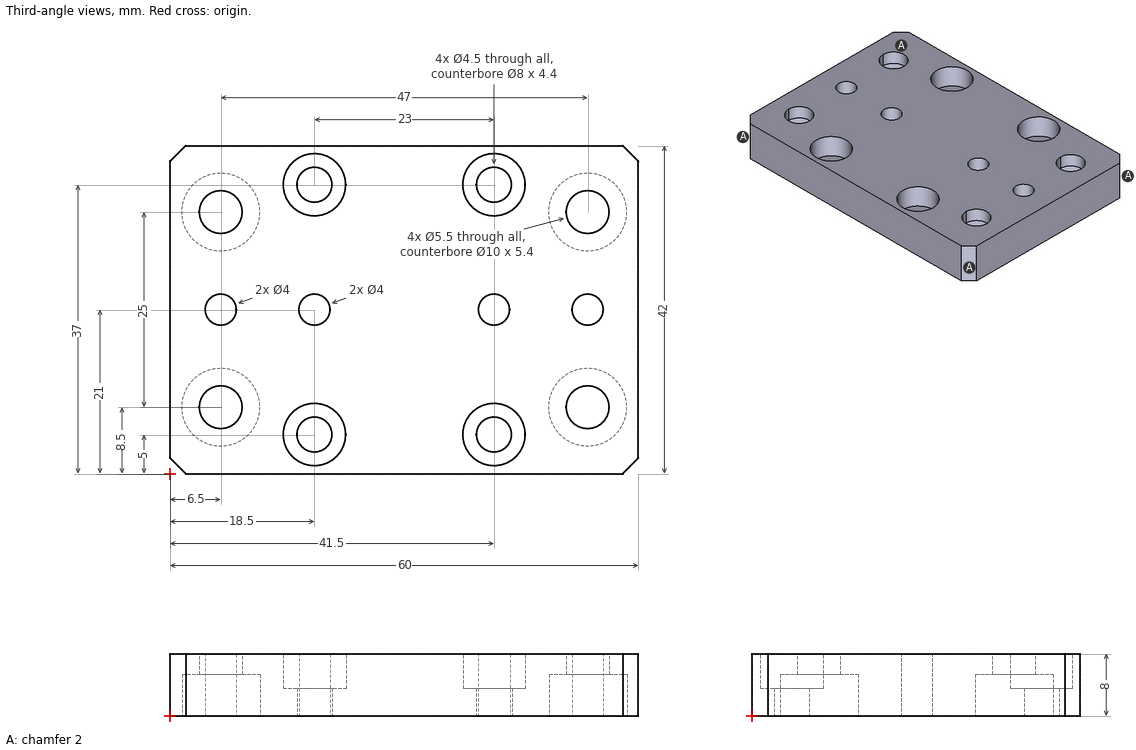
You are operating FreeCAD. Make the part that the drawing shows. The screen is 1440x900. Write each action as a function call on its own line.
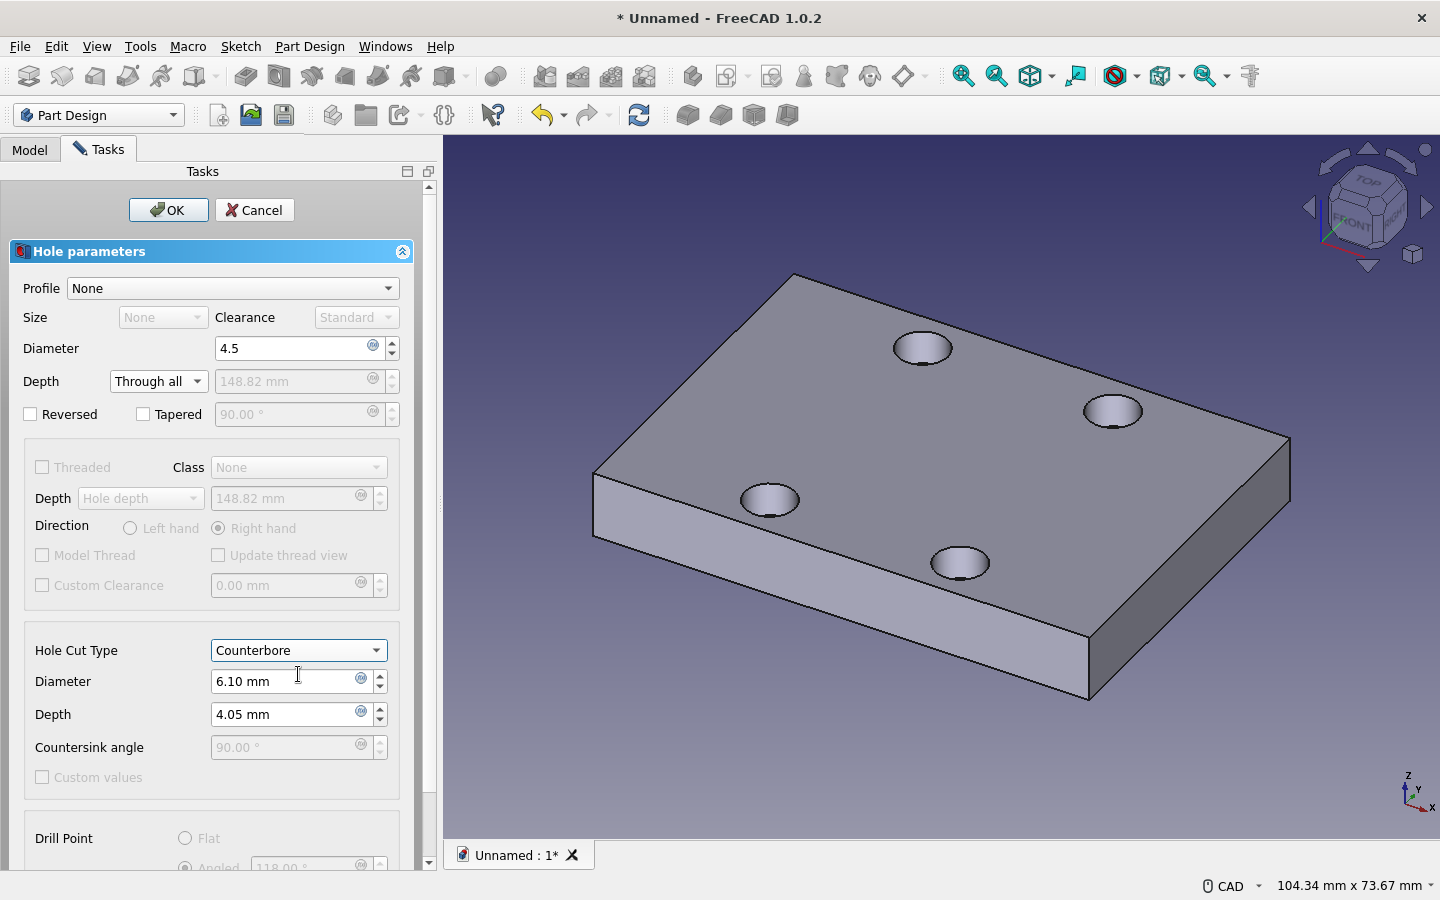
triple_click(292, 682)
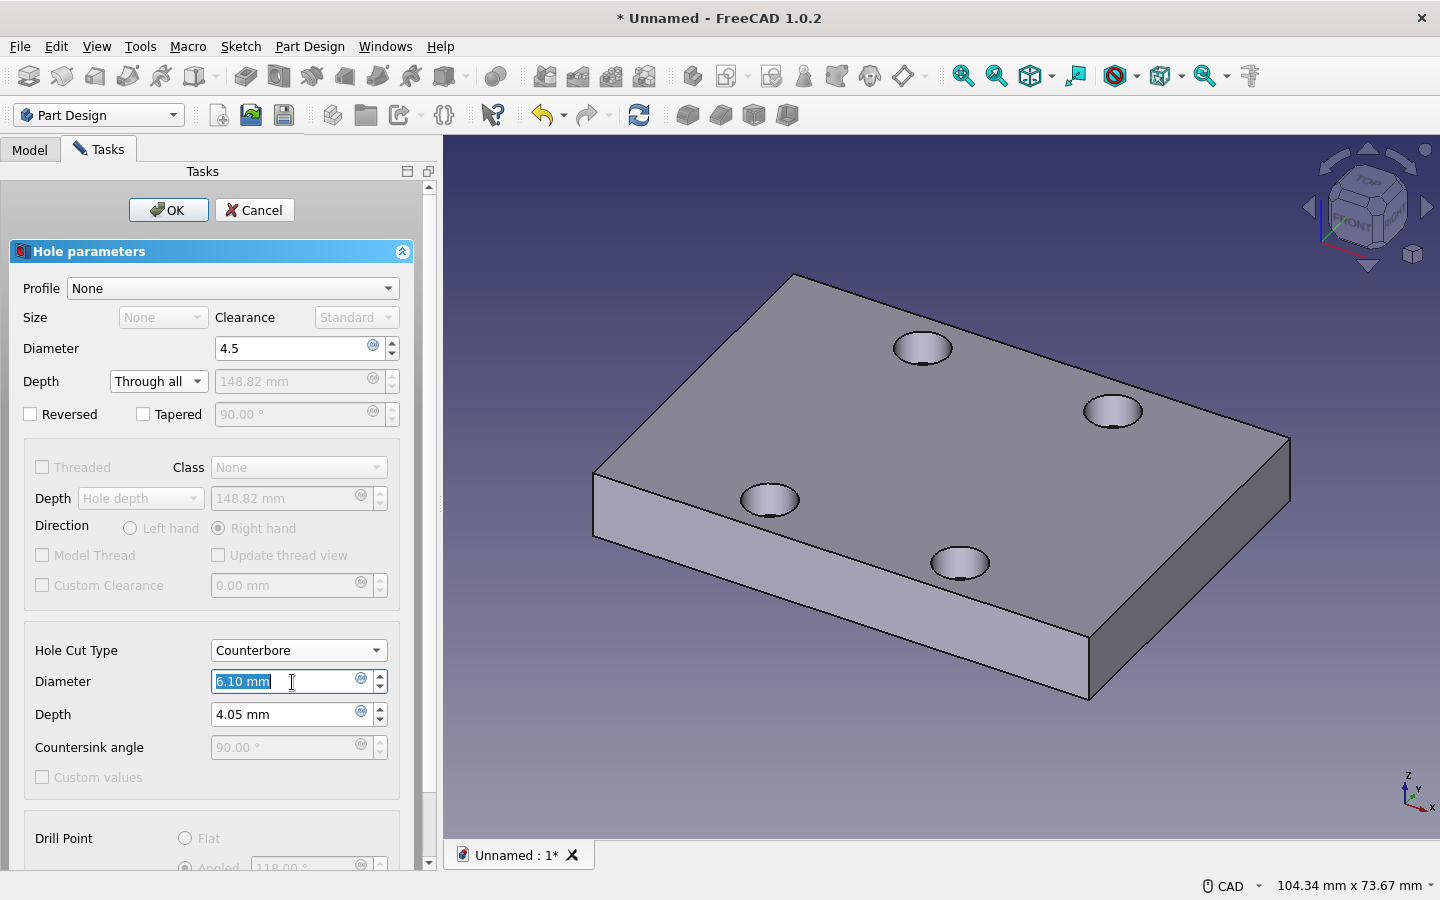
text(8)
key(Tab)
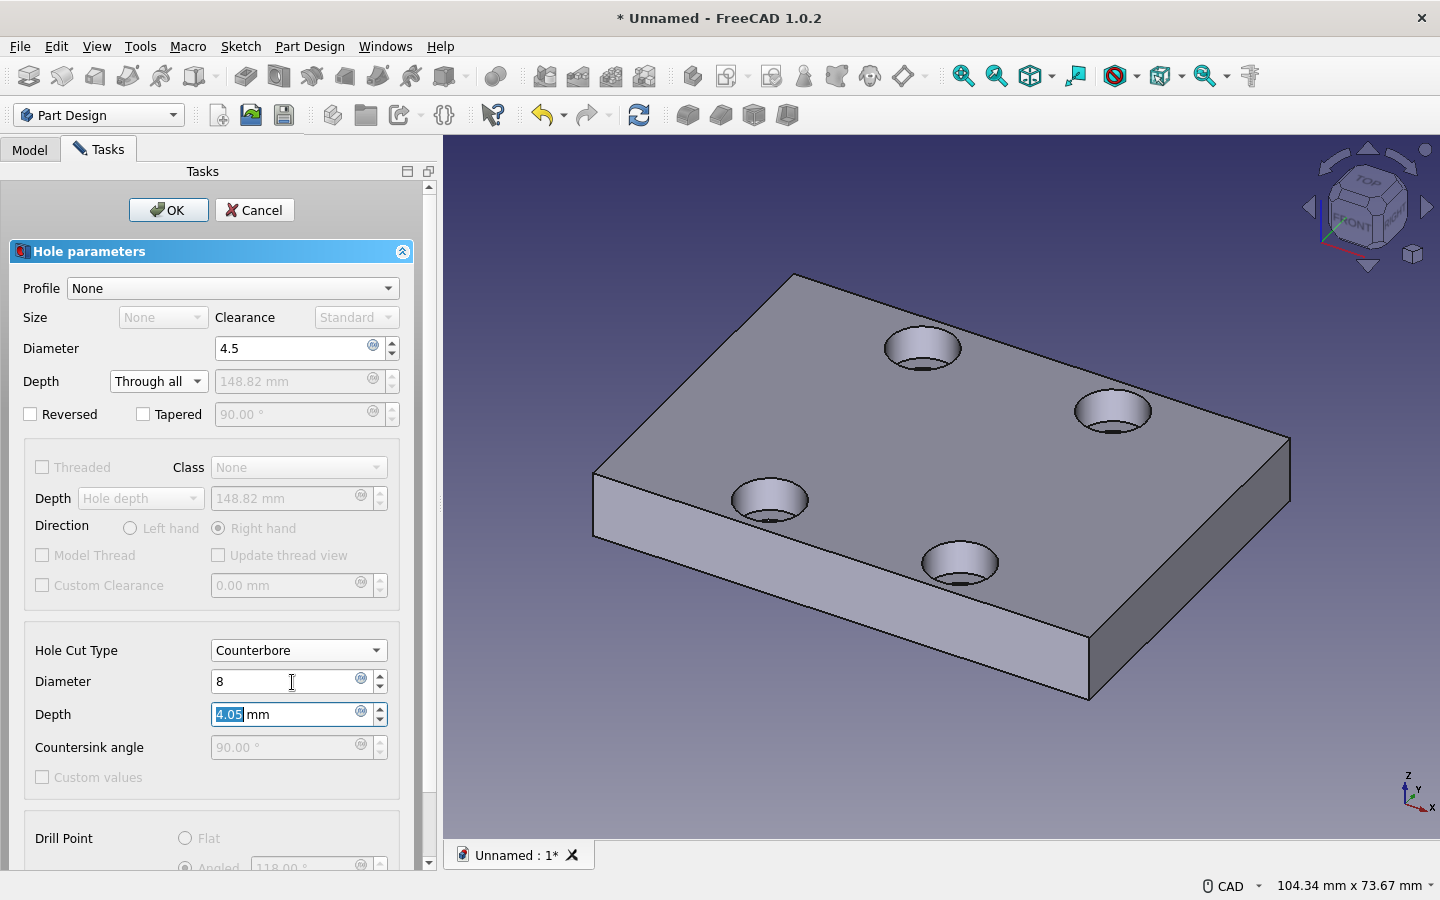
text(4.4)
key(Tab)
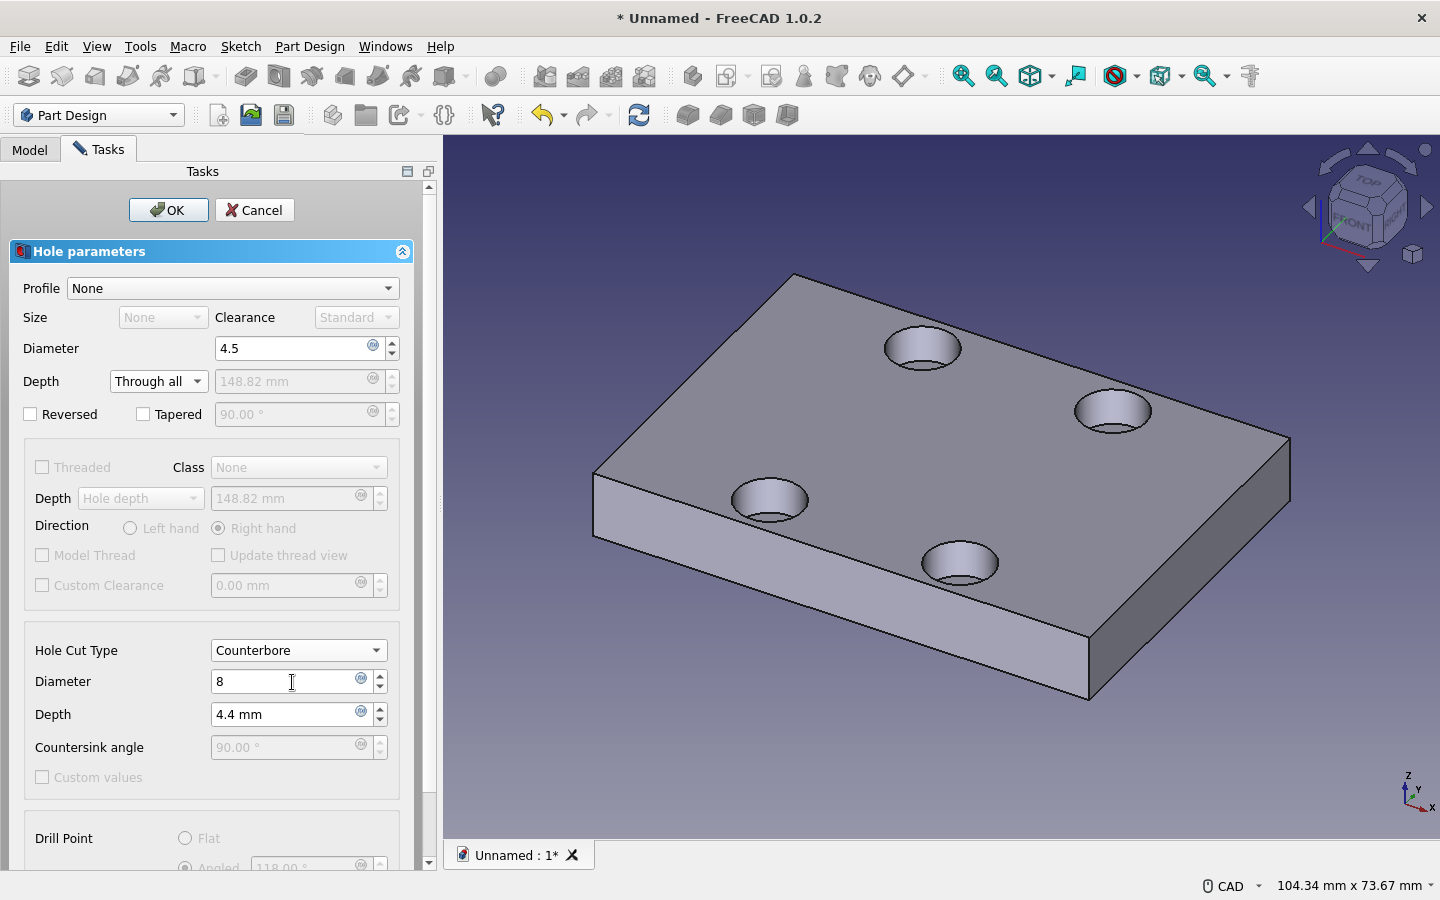
click(169, 210)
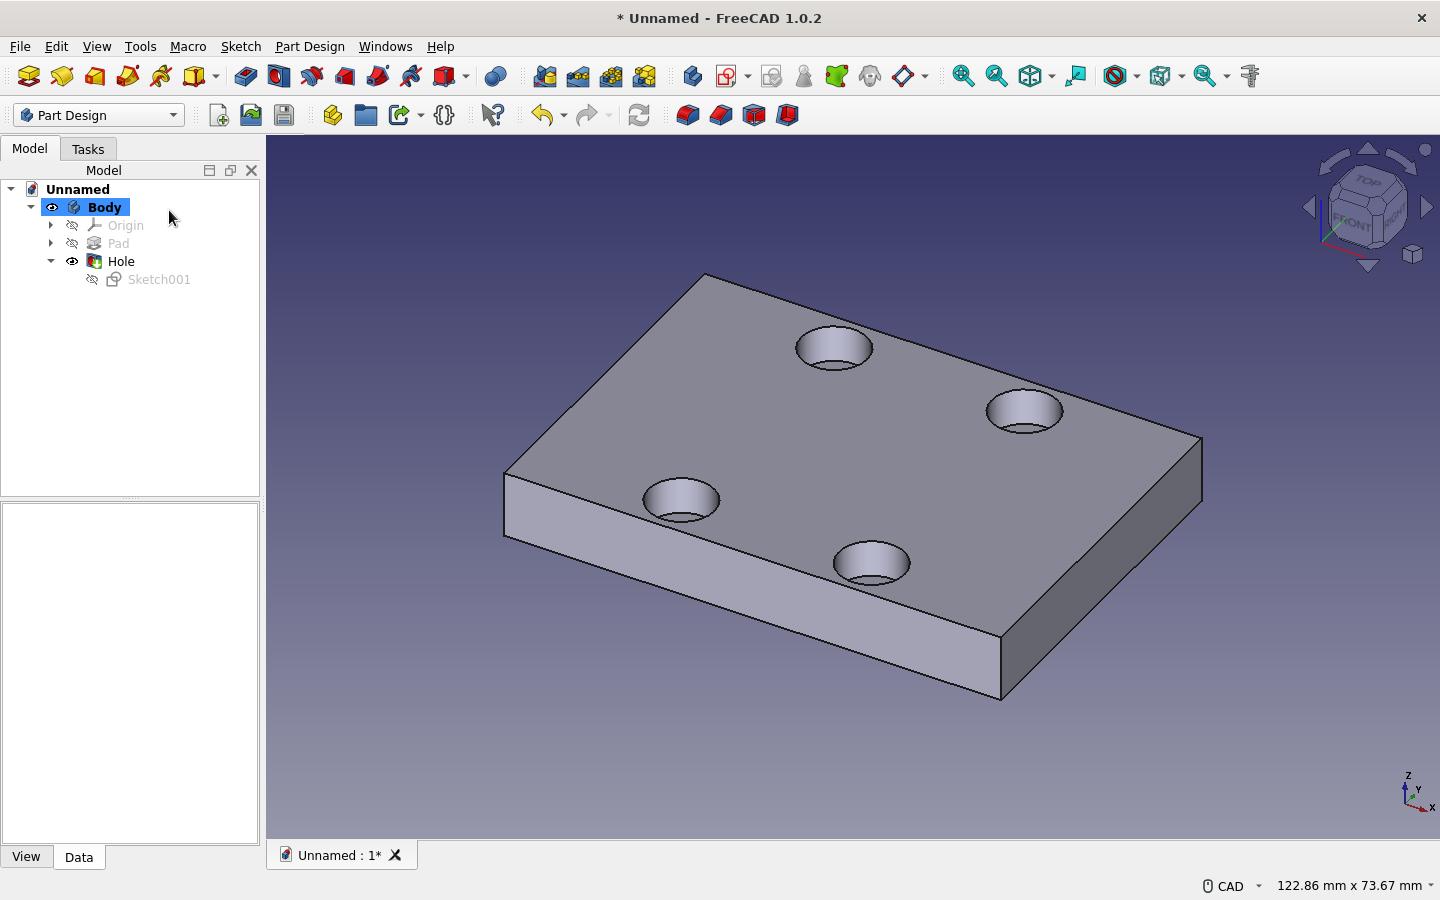
click(853, 455)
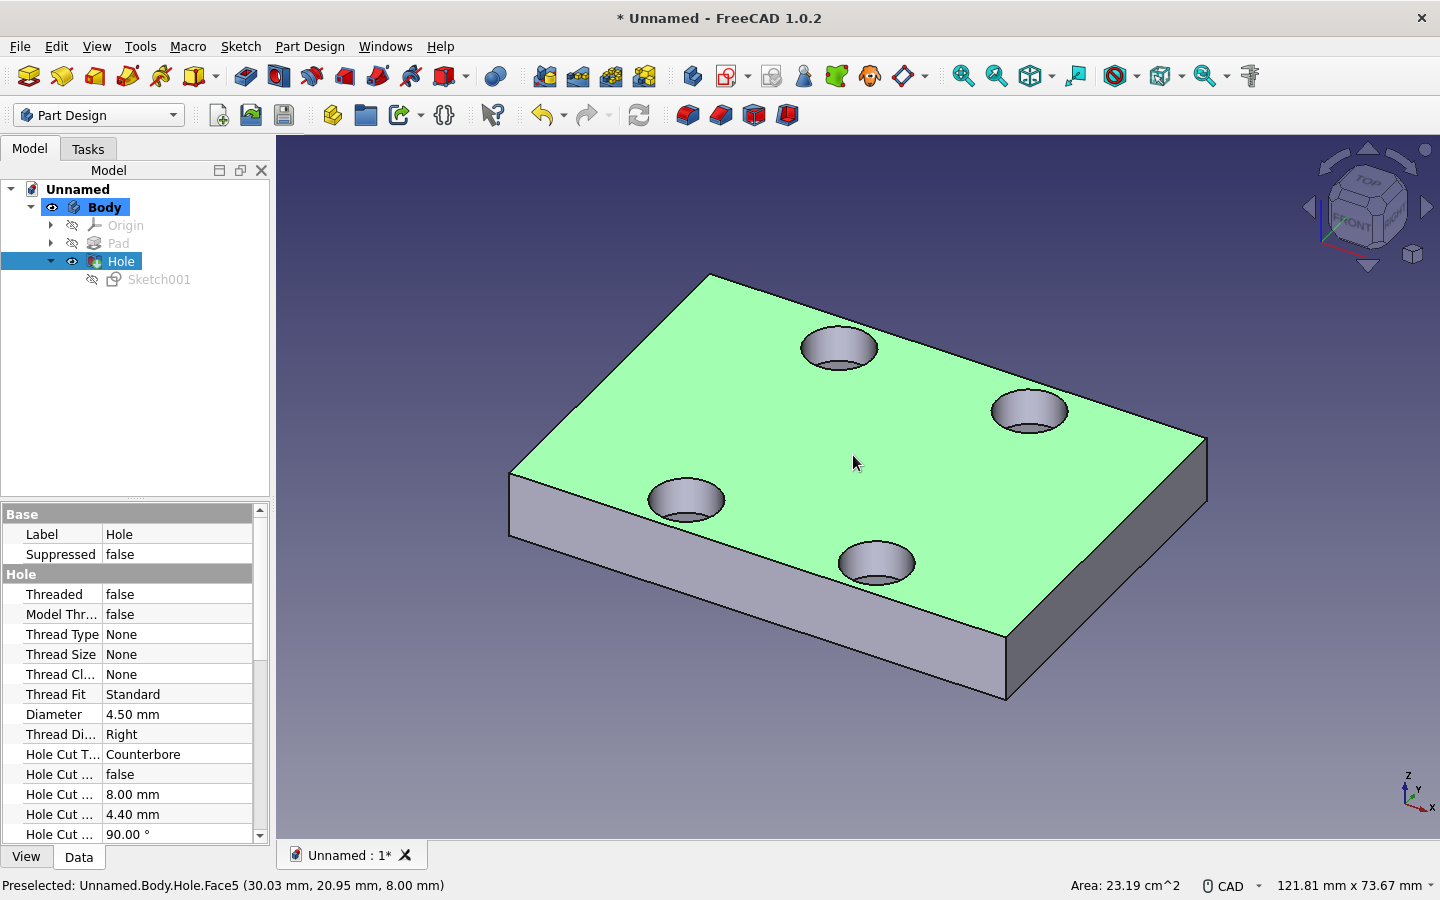
click(726, 76)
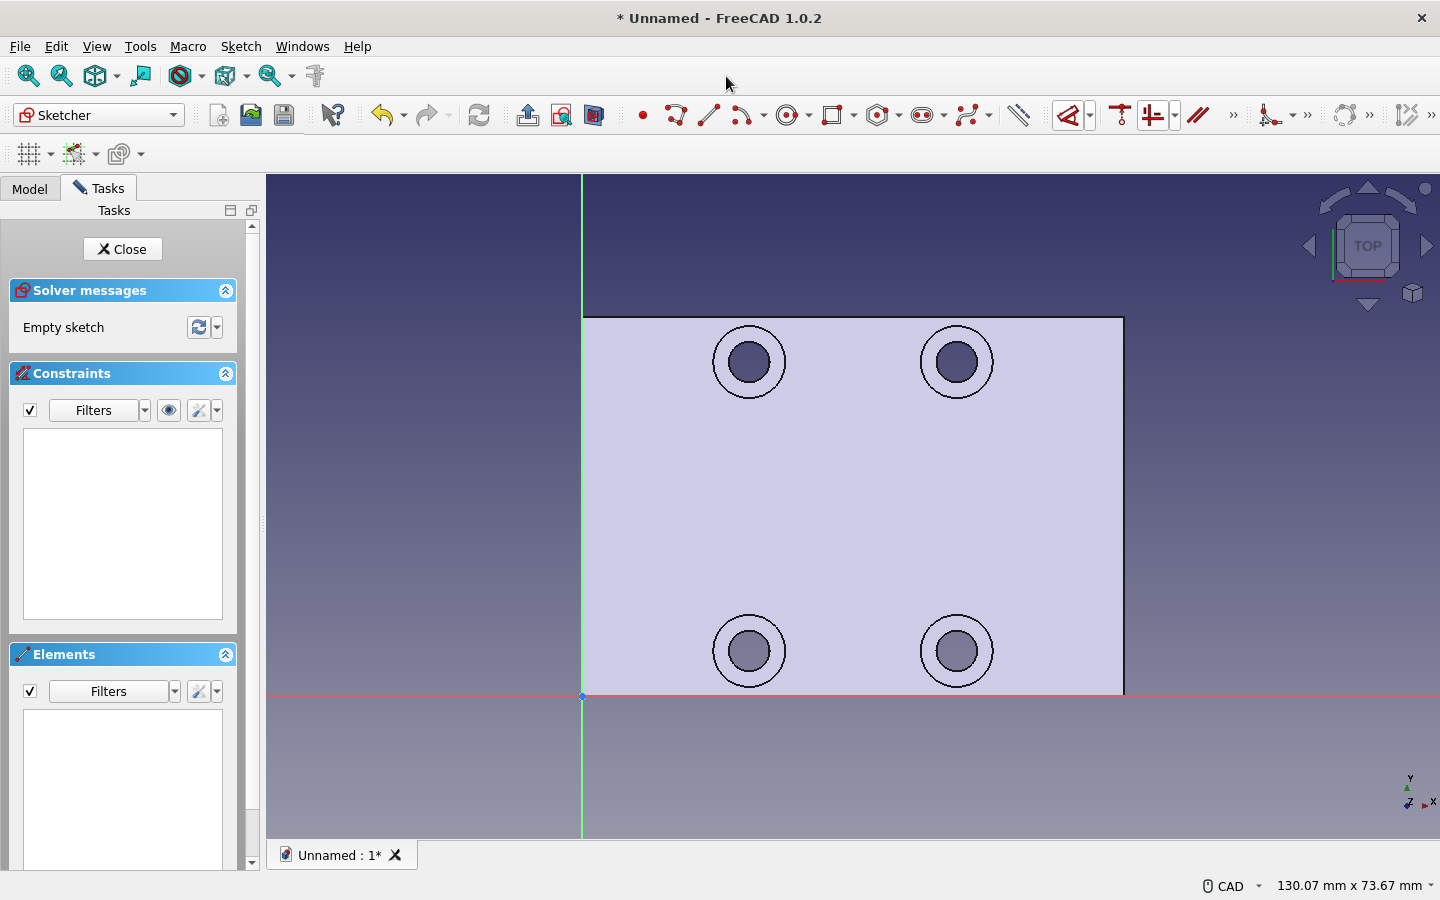
scroll(771, 697, up, 3)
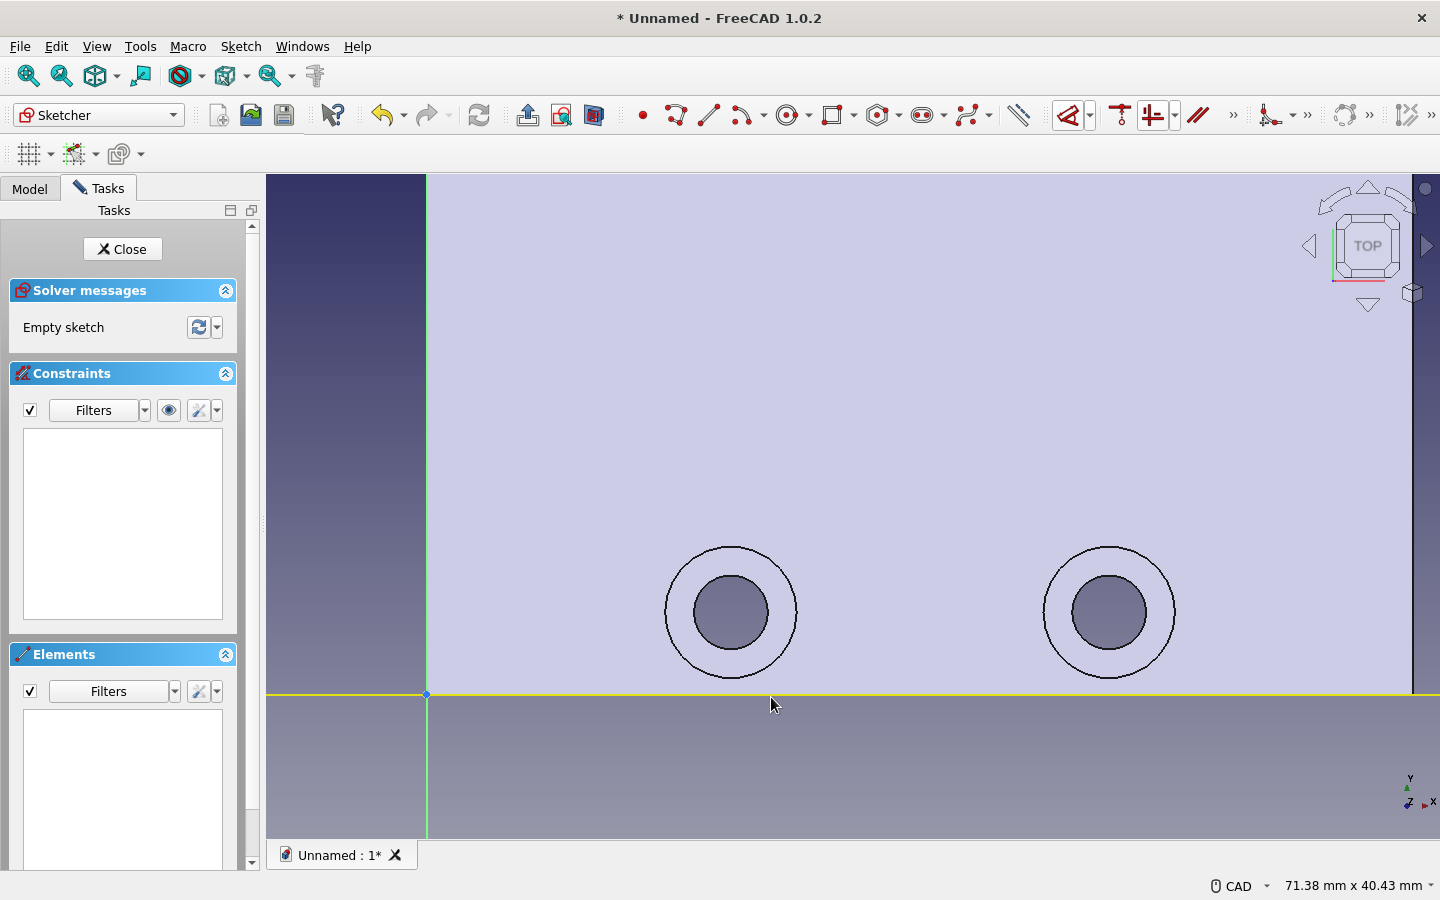
click(786, 116)